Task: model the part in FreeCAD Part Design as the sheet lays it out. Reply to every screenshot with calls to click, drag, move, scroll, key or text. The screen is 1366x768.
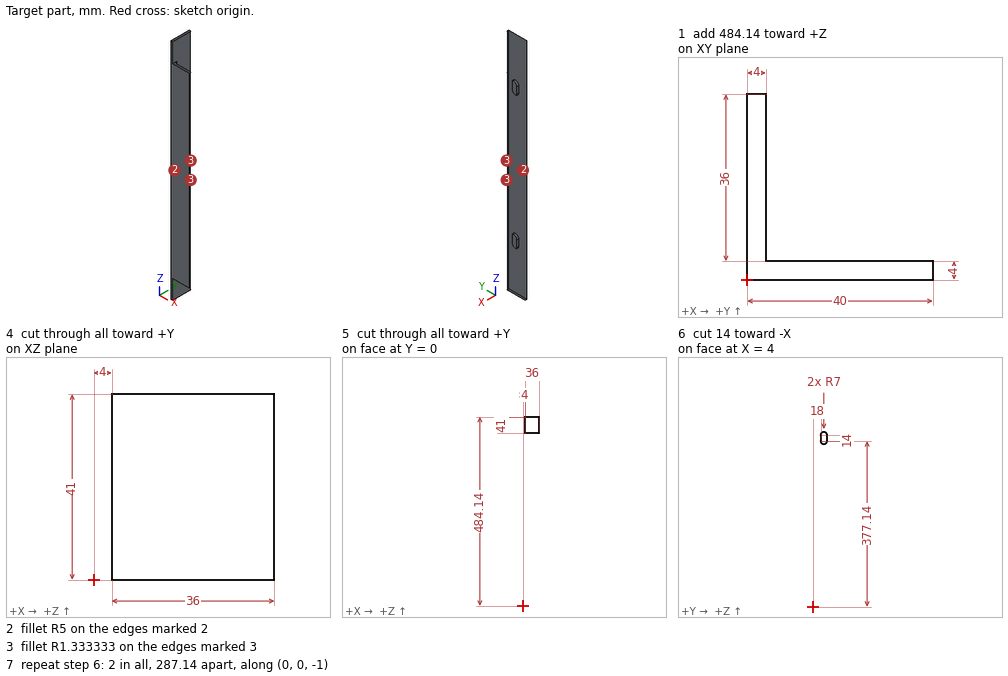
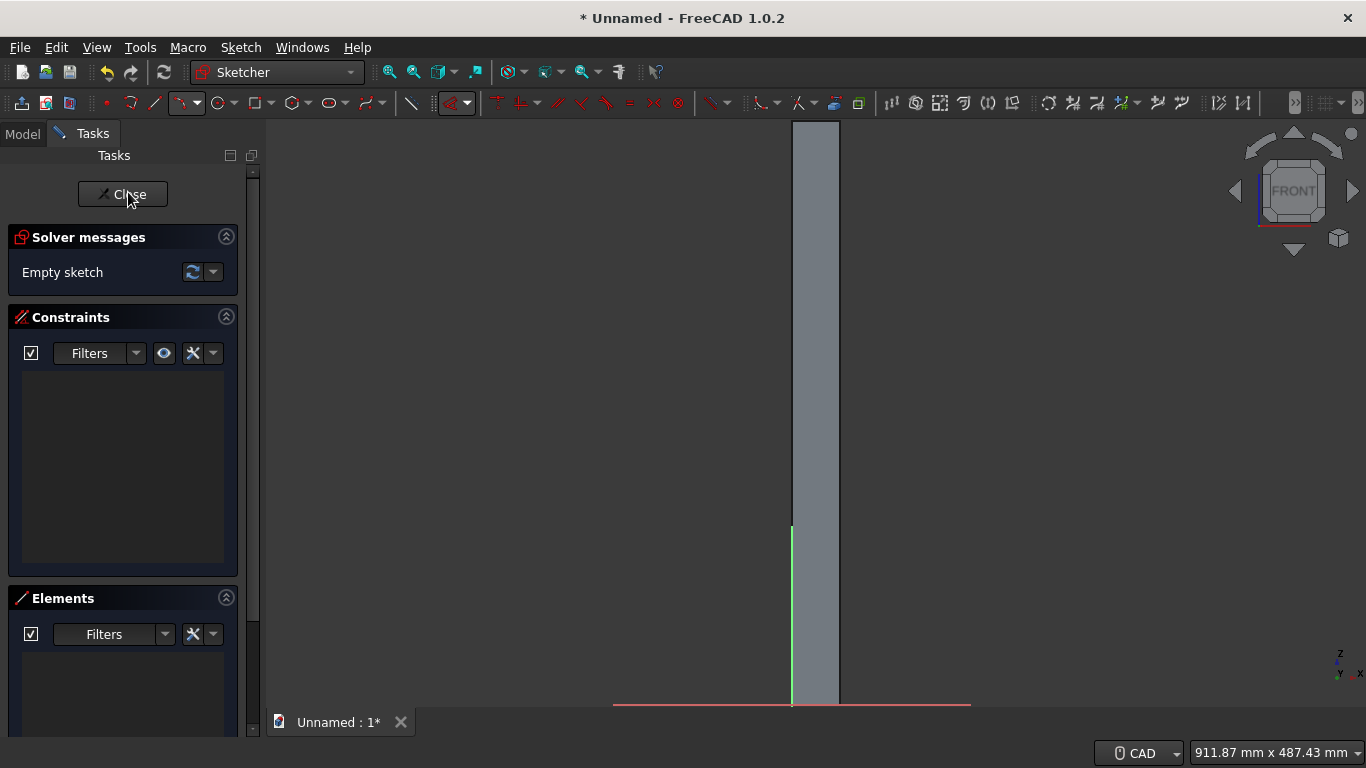
scroll(748, 413, down, 5)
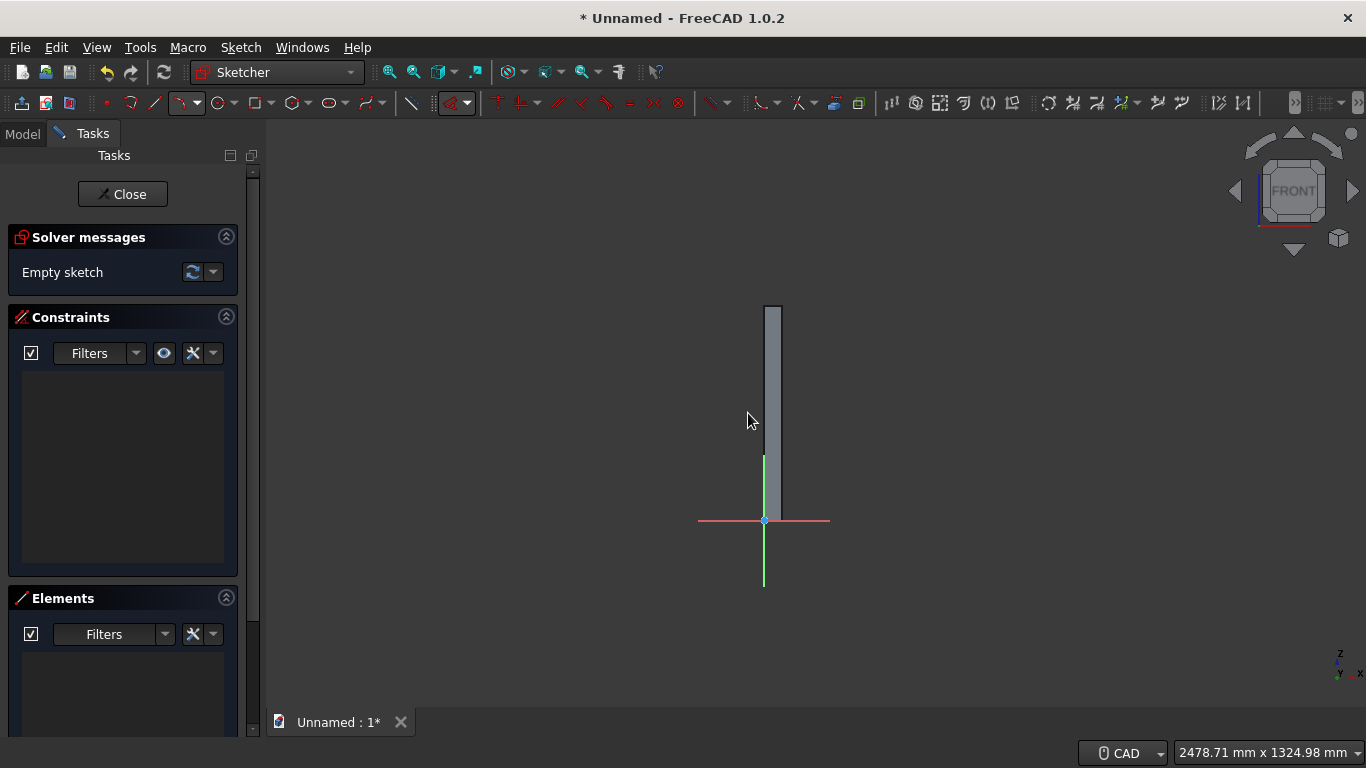
scroll(775, 517, up, 15)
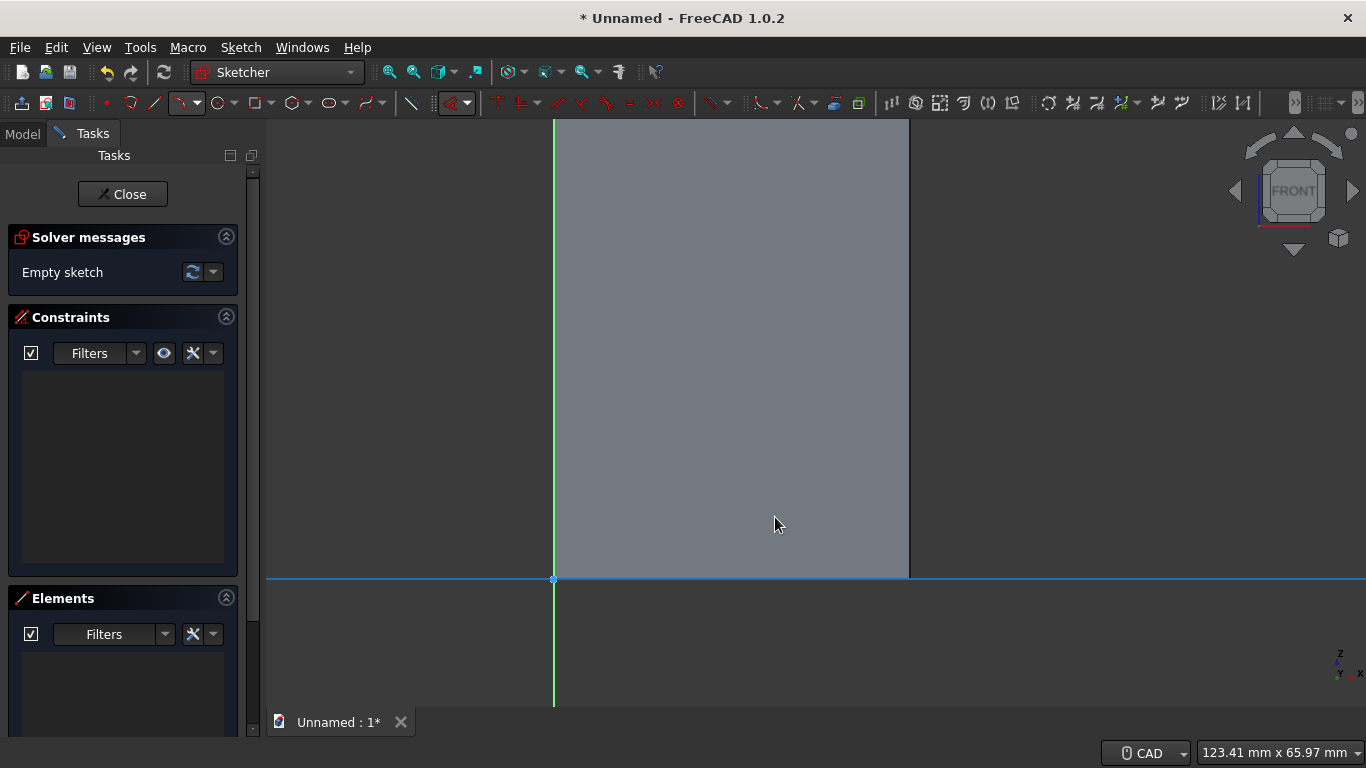
click(256, 104)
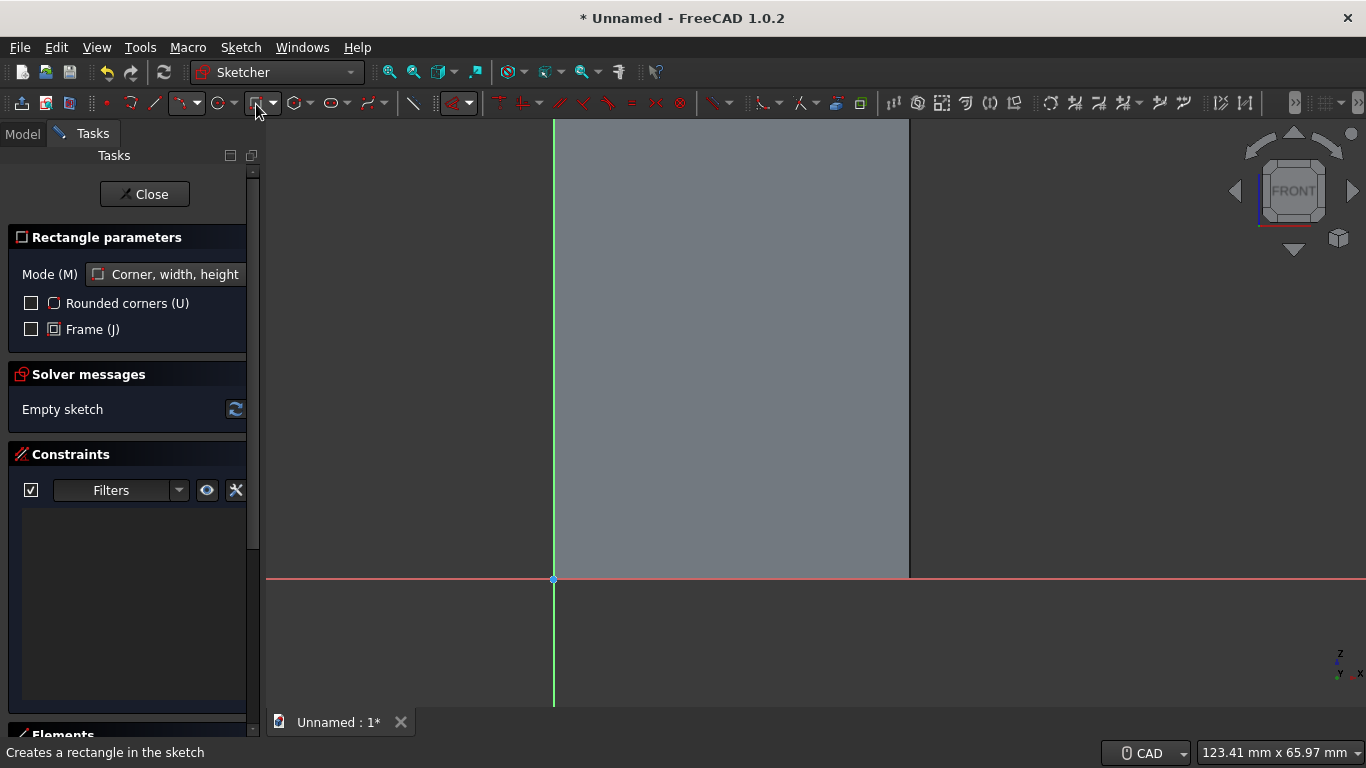
click(589, 214)
click(910, 579)
key(Escape)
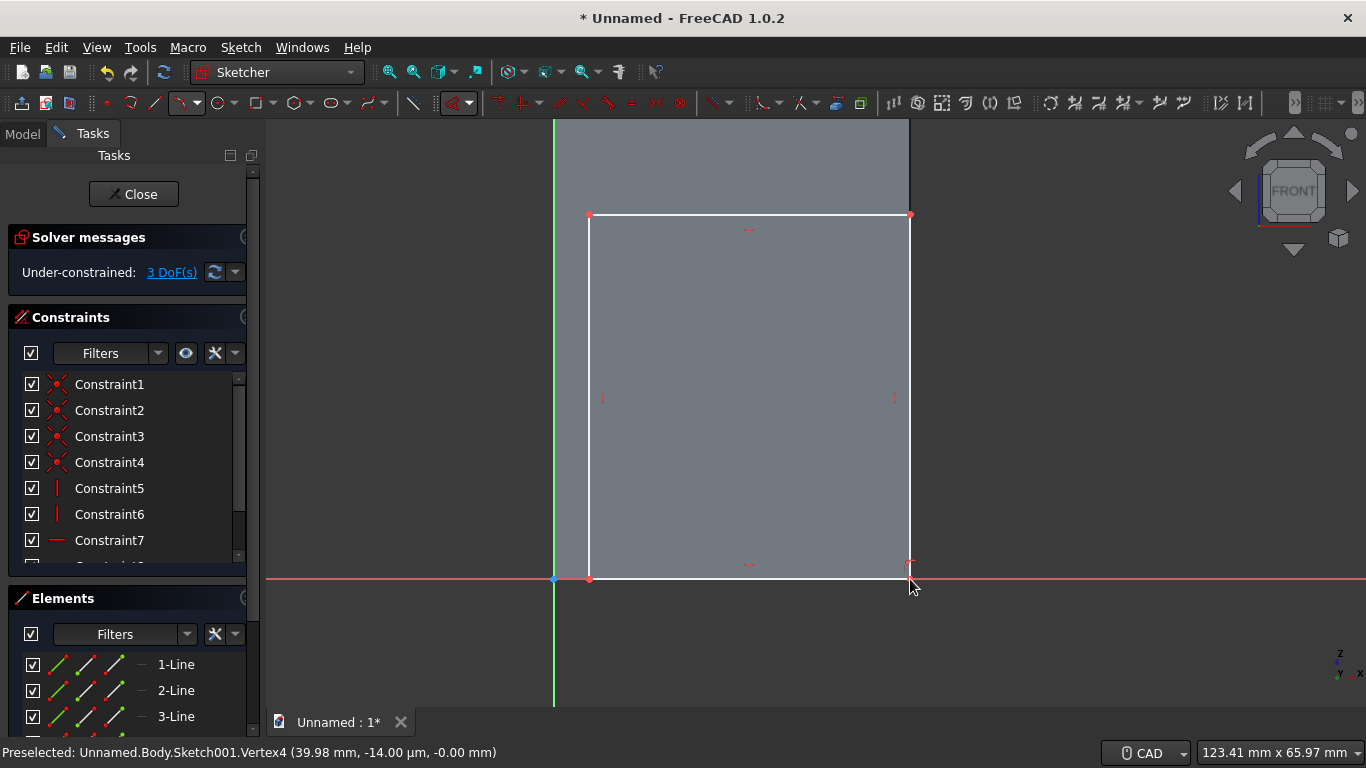
click(589, 324)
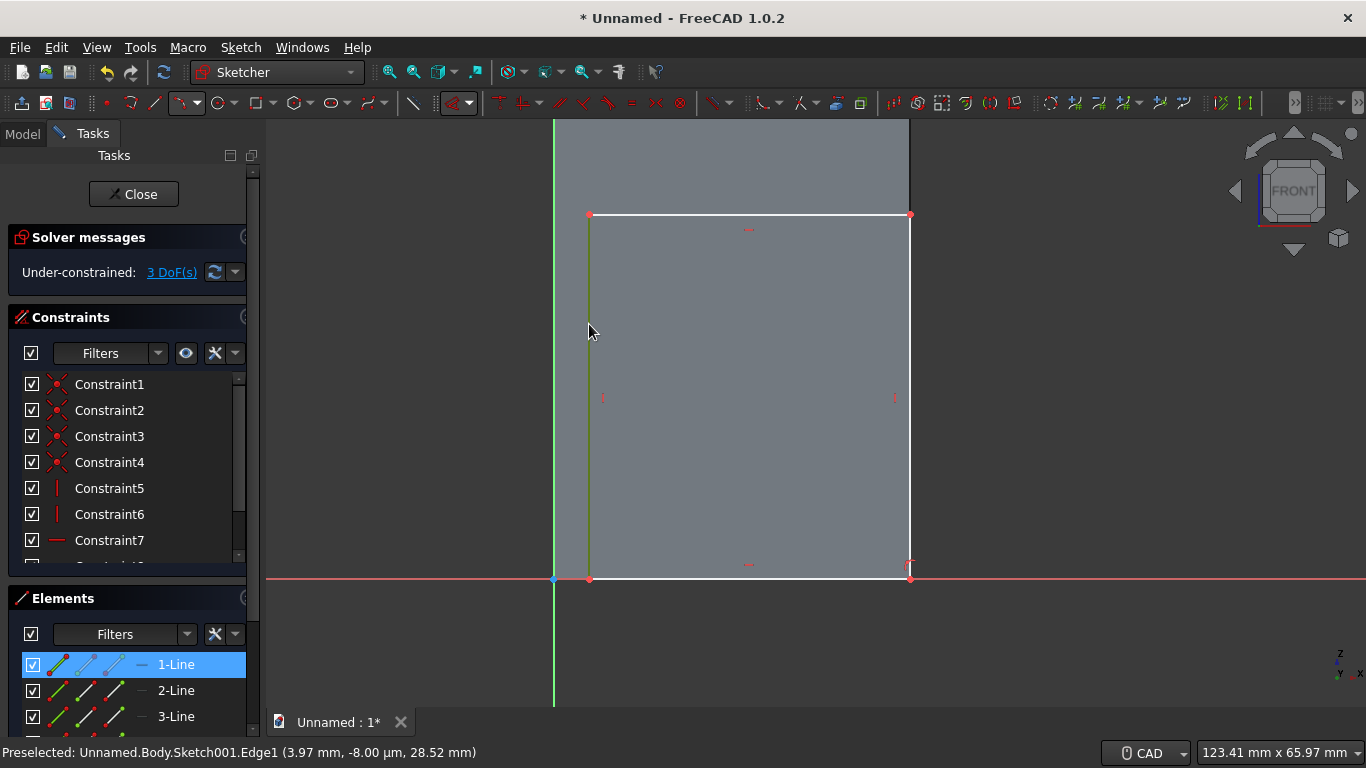
click(472, 104)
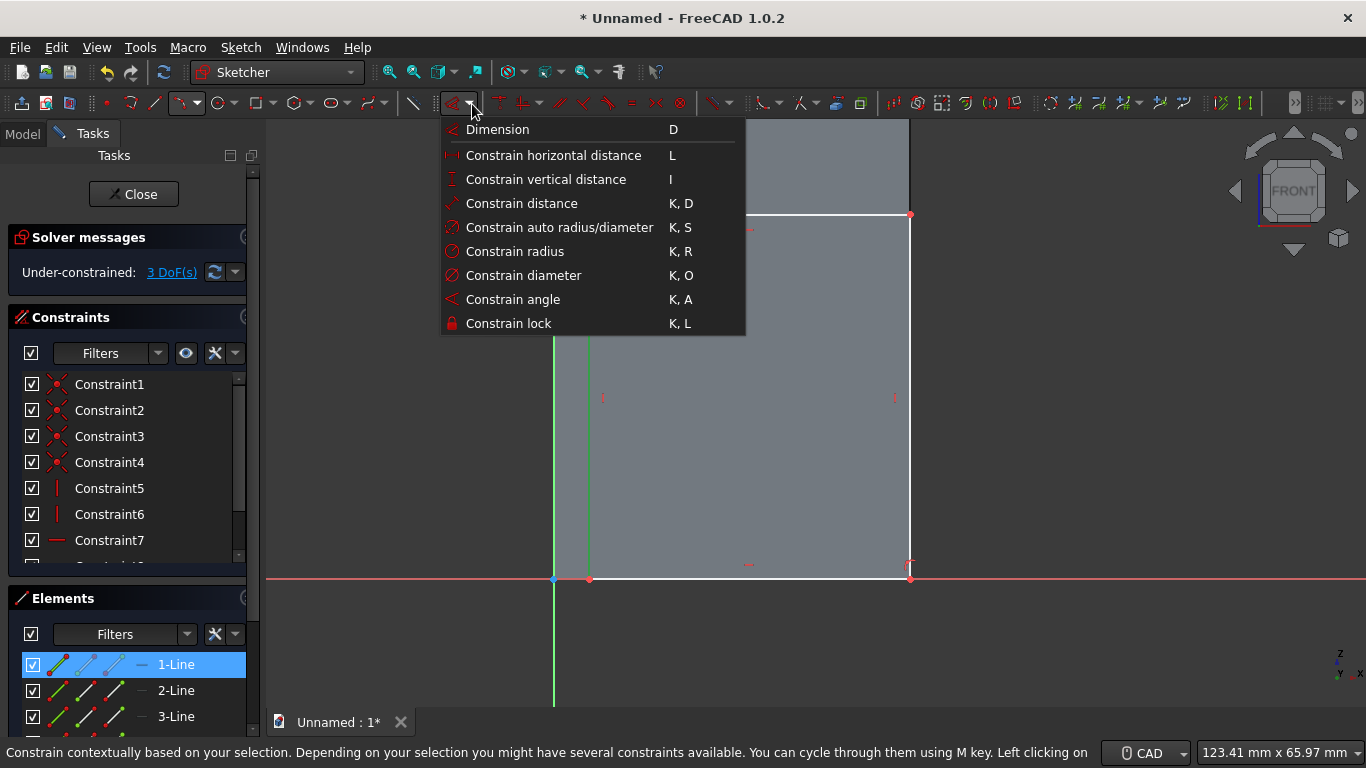
click(593, 179)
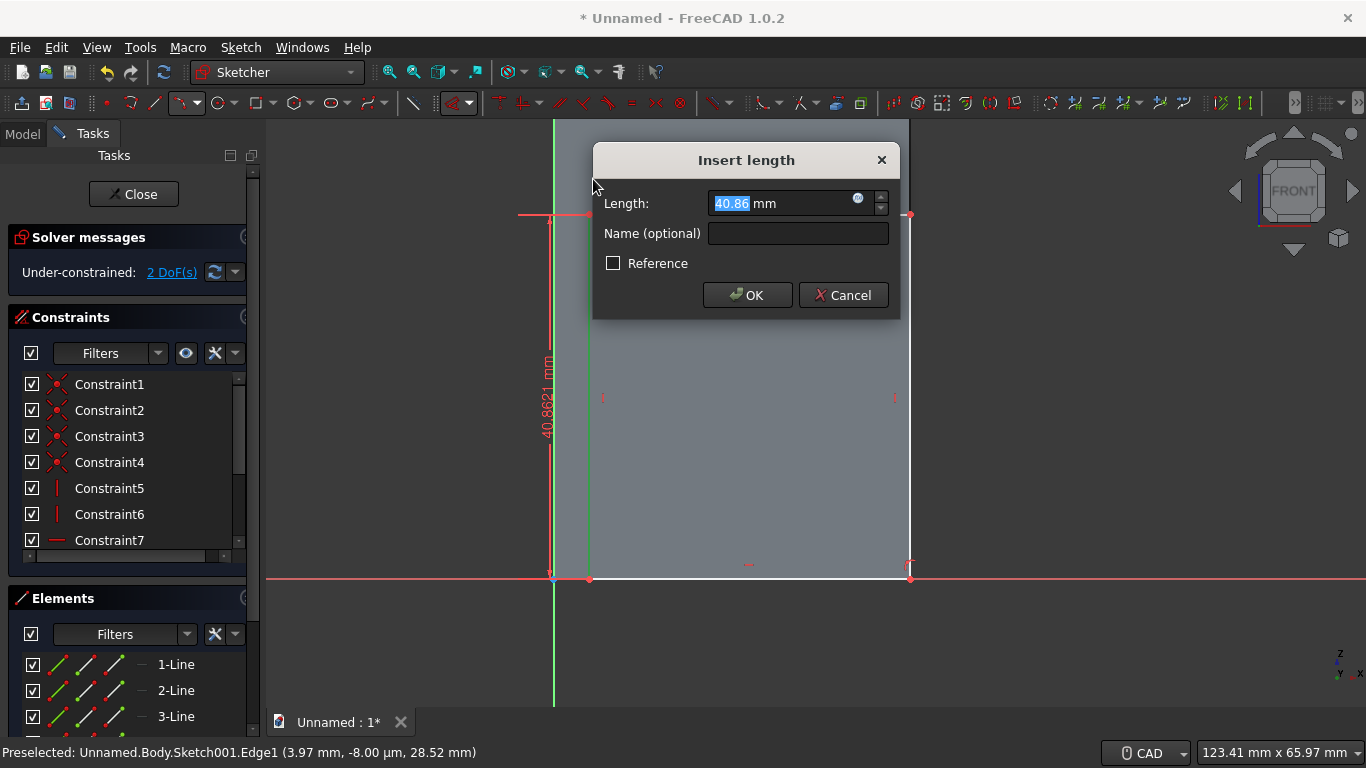
text(41)
key(Return)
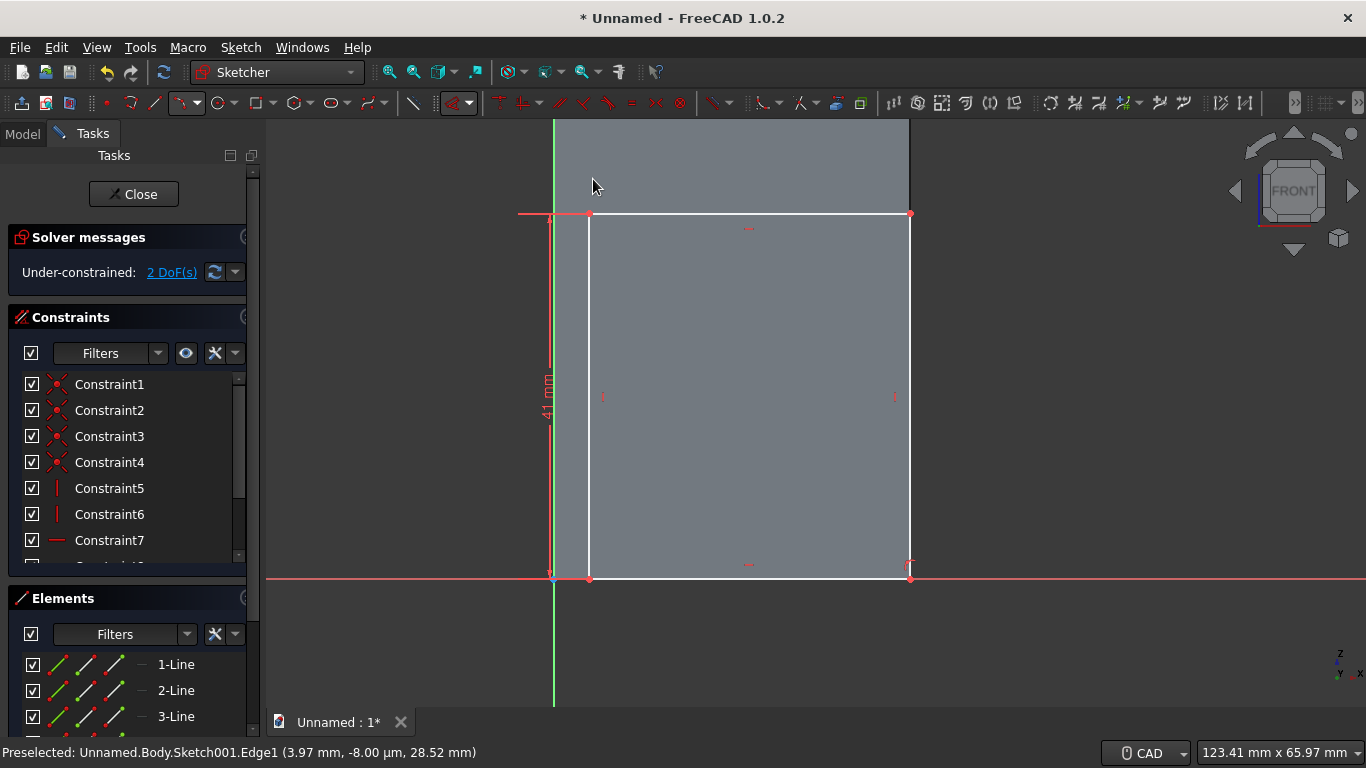
click(685, 579)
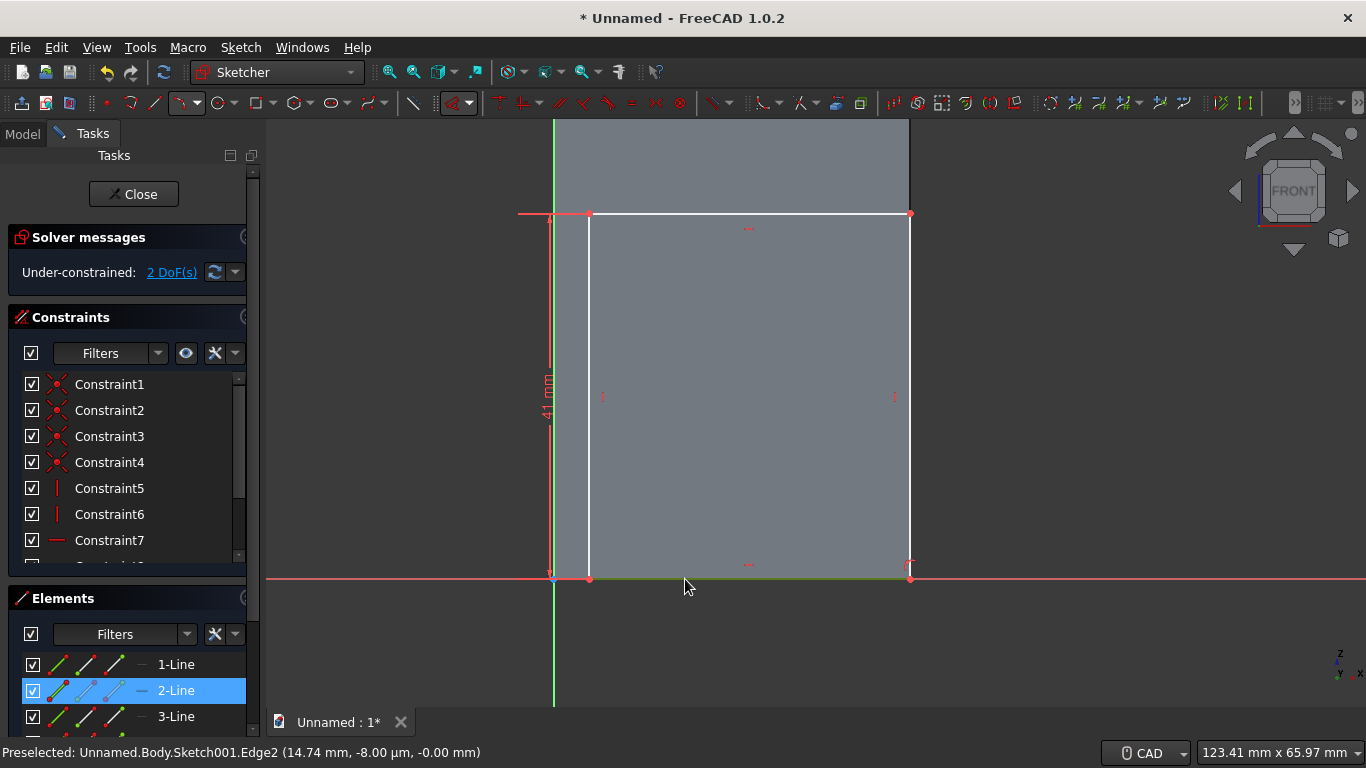
key(l)